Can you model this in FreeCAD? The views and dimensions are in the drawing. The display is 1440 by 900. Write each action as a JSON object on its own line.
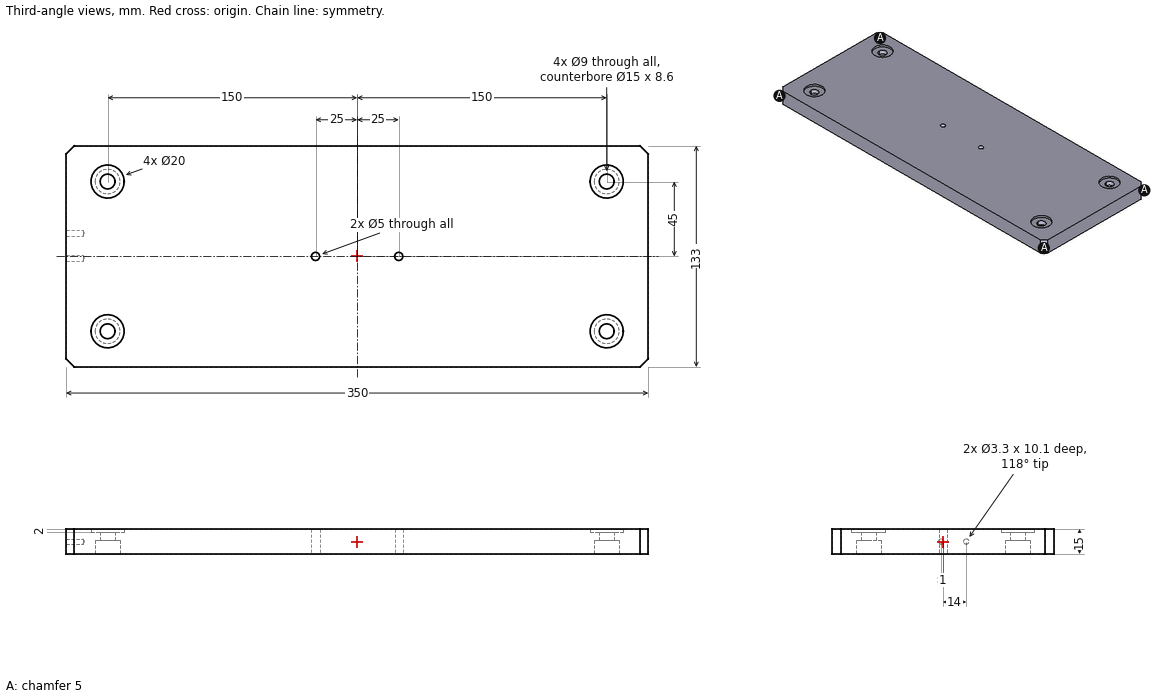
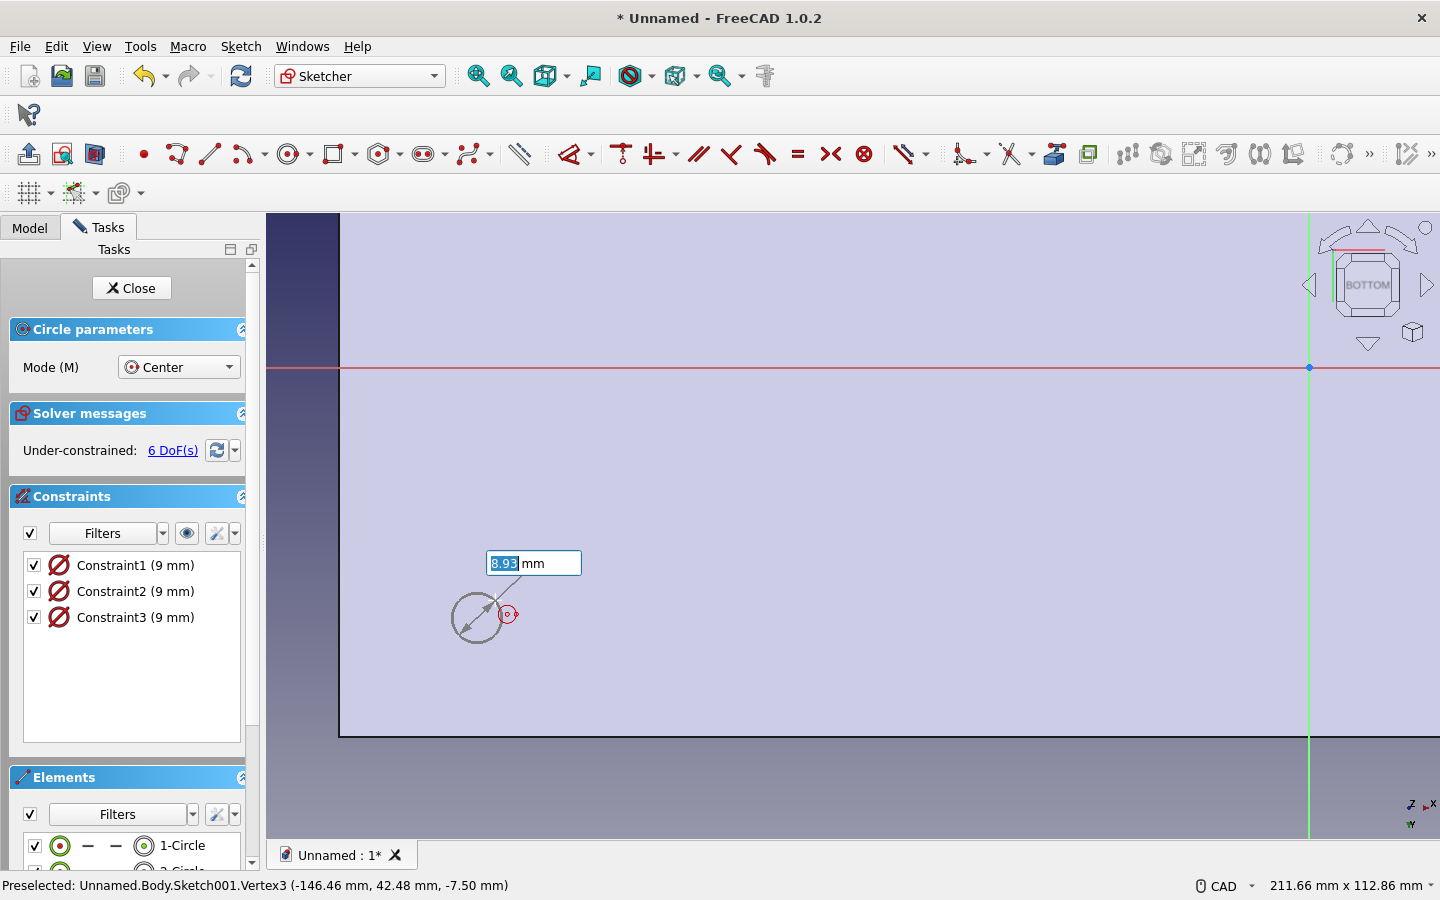
{"action": "type", "text": "9"}
{"action": "key", "text": "Return"}
{"action": "key", "text": "Escape"}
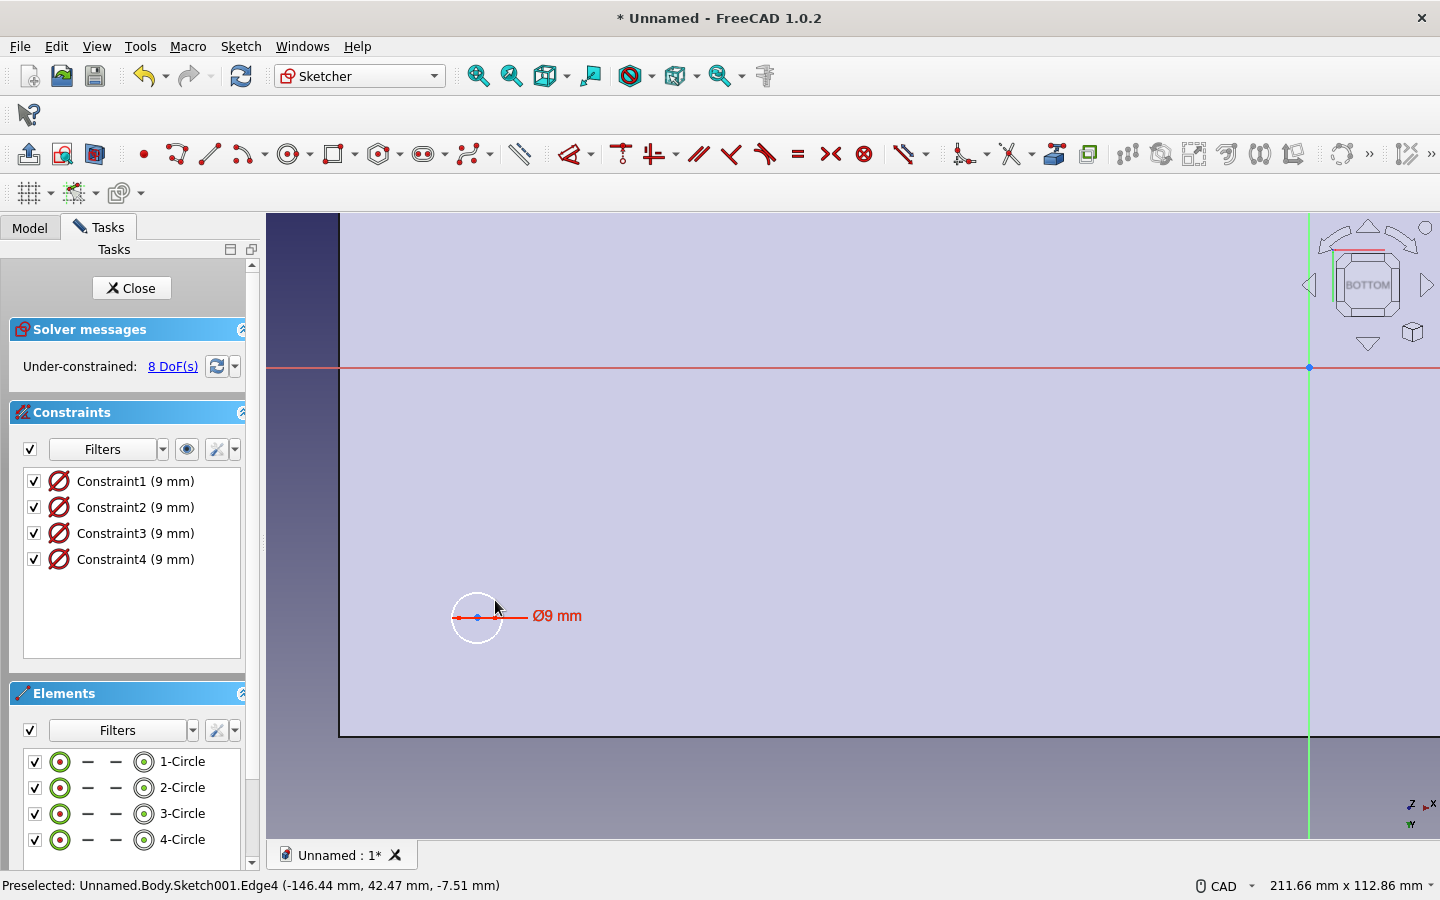
{"action": "scroll", "coordinate": [479, 618], "scroll_direction": "down", "scroll_amount": 5}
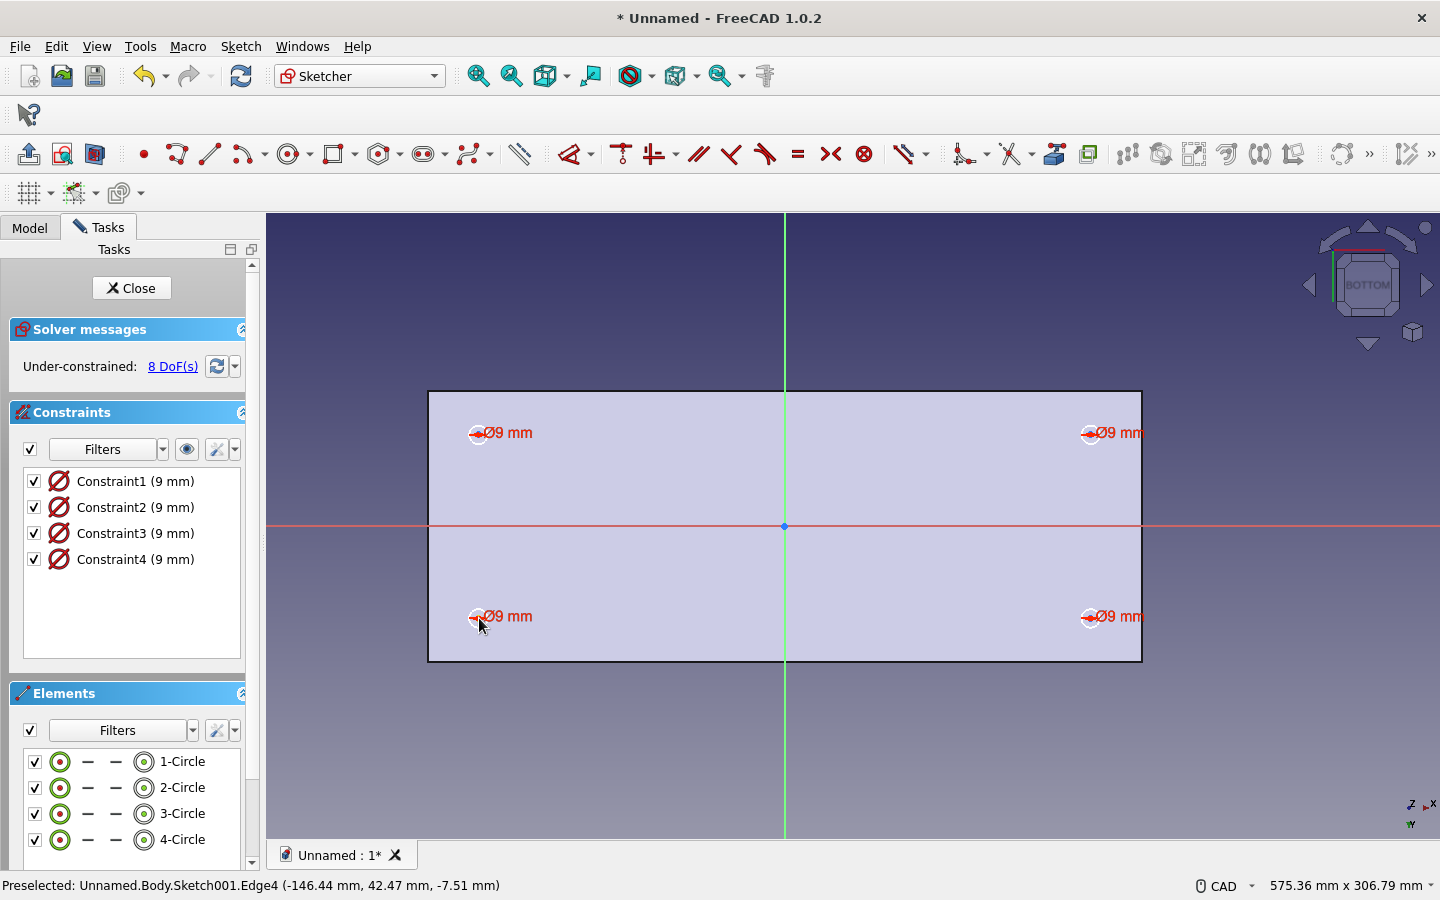
{"action": "left_click", "coordinate": [1091, 618]}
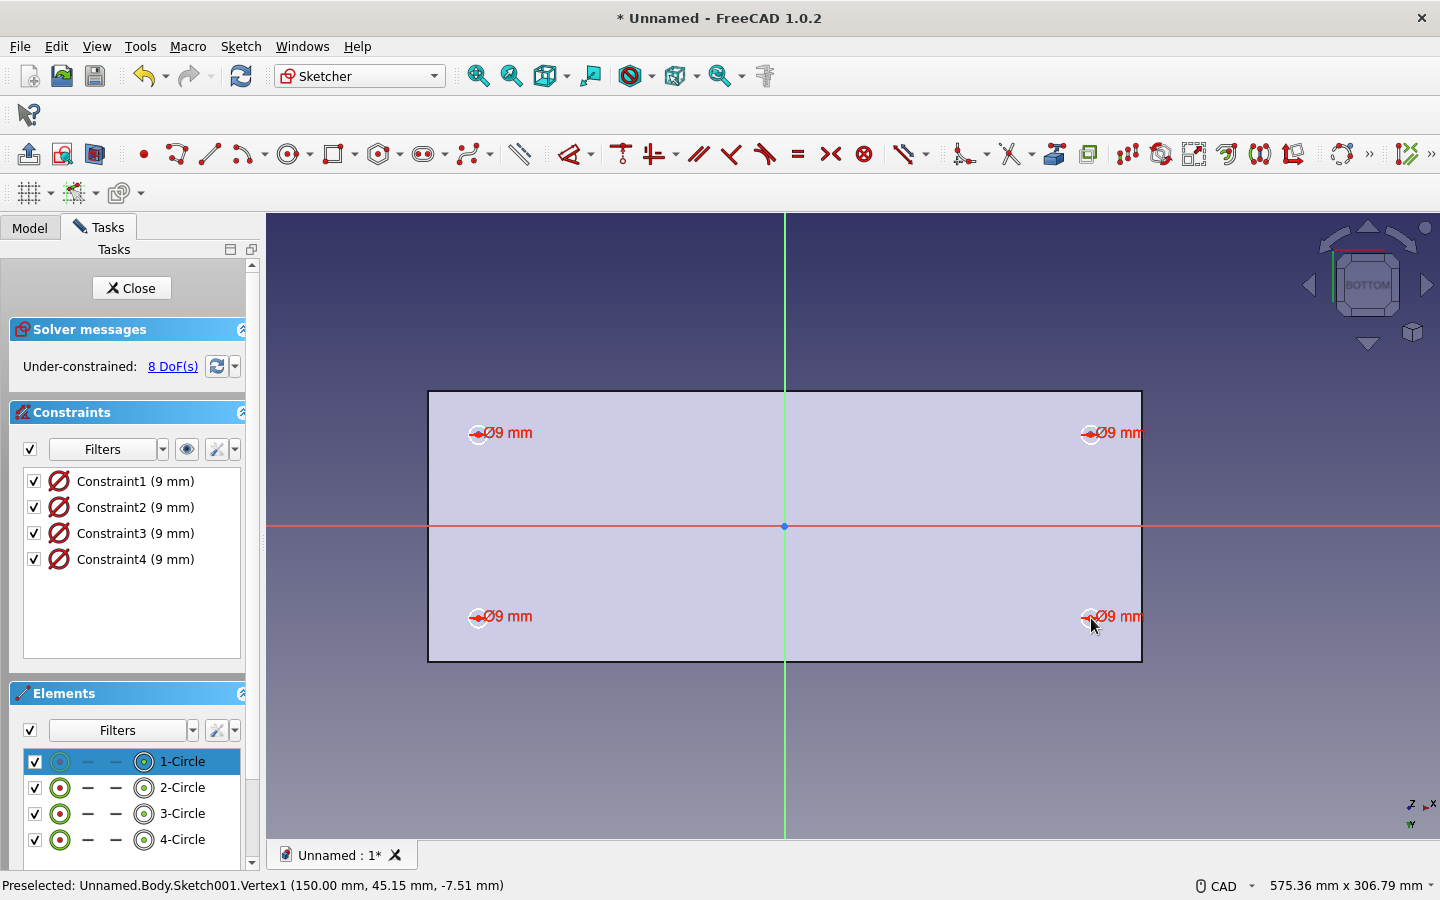
{"action": "left_click", "coordinate": [1091, 435]}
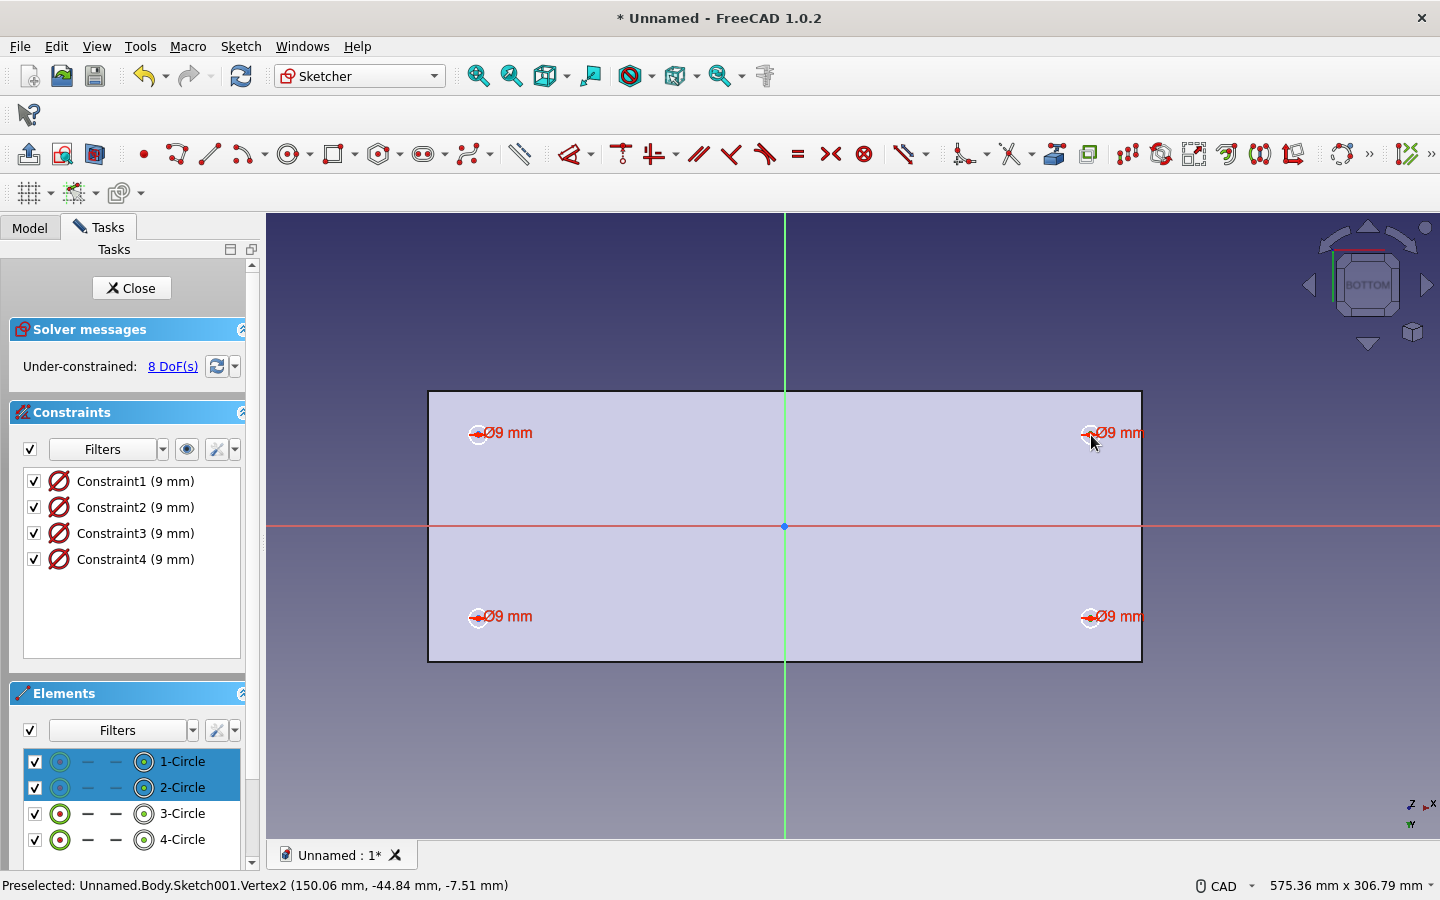
{"action": "left_click", "coordinate": [364, 526]}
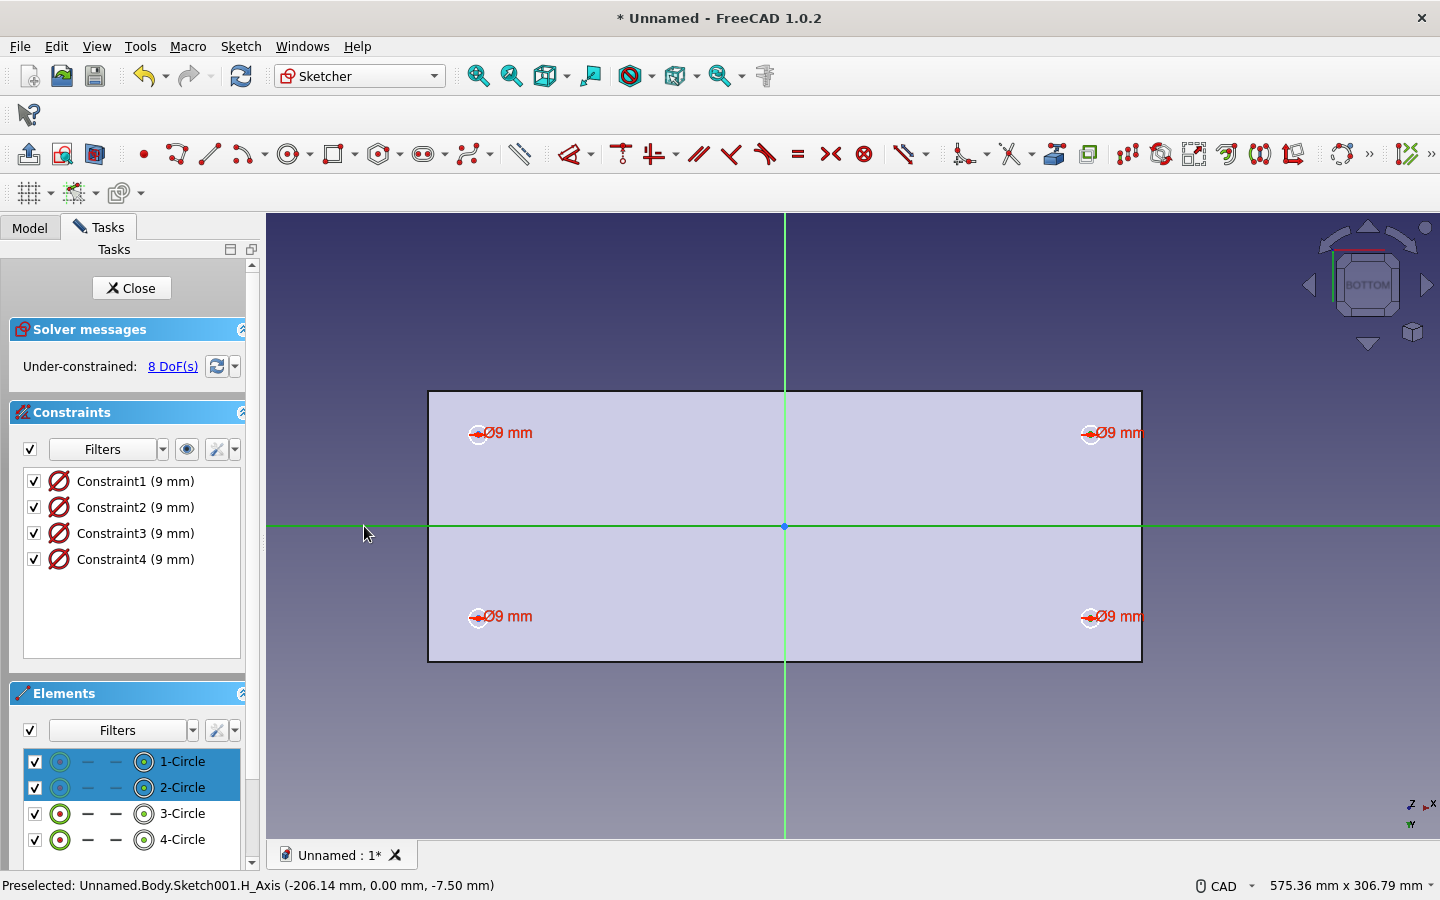
{"action": "key", "text": "s"}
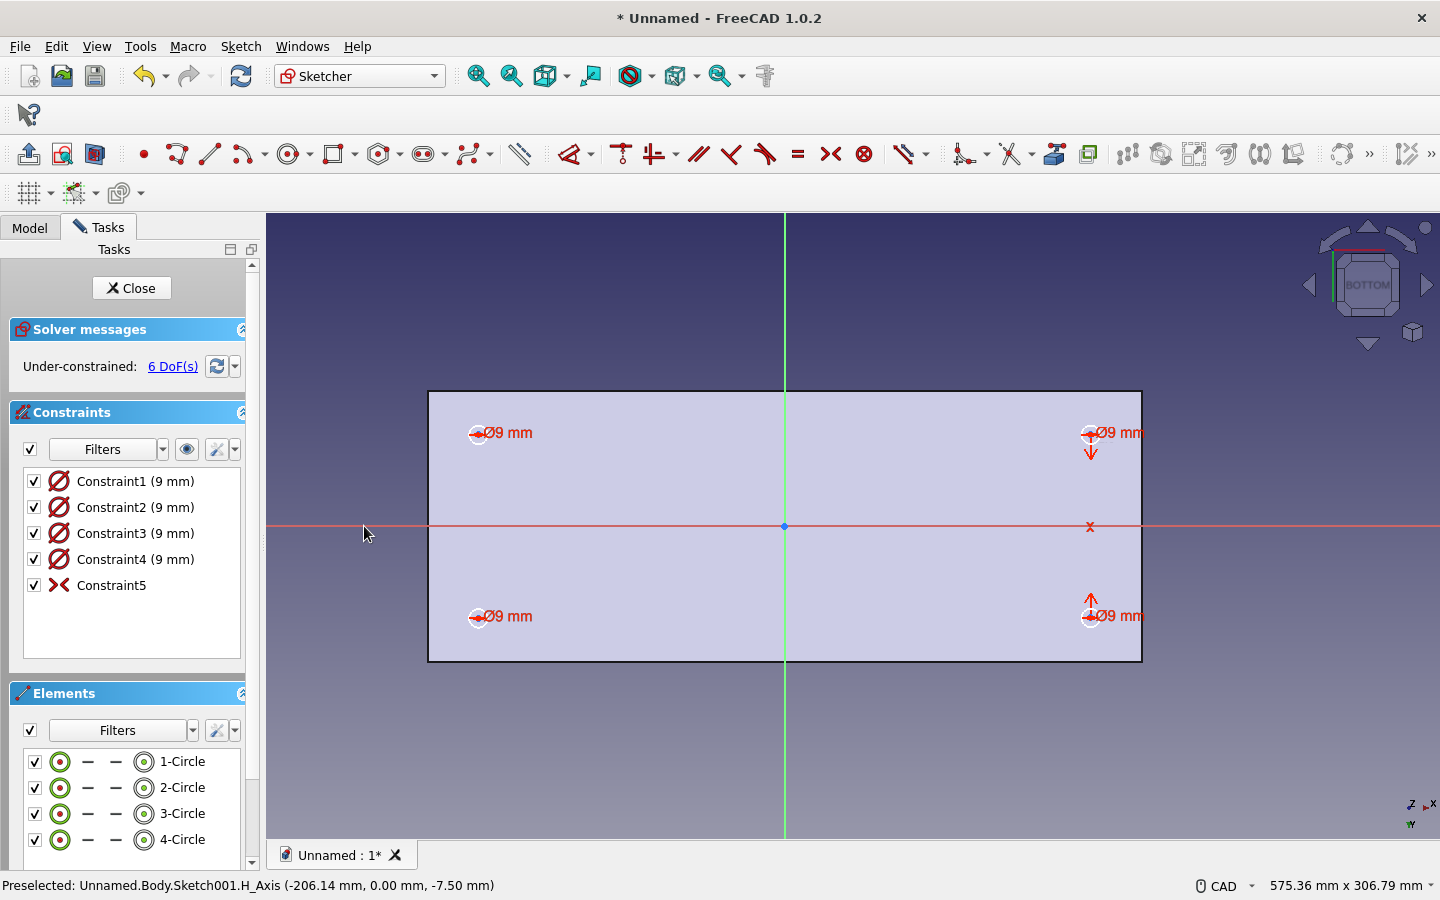
{"action": "left_click", "coordinate": [1091, 435]}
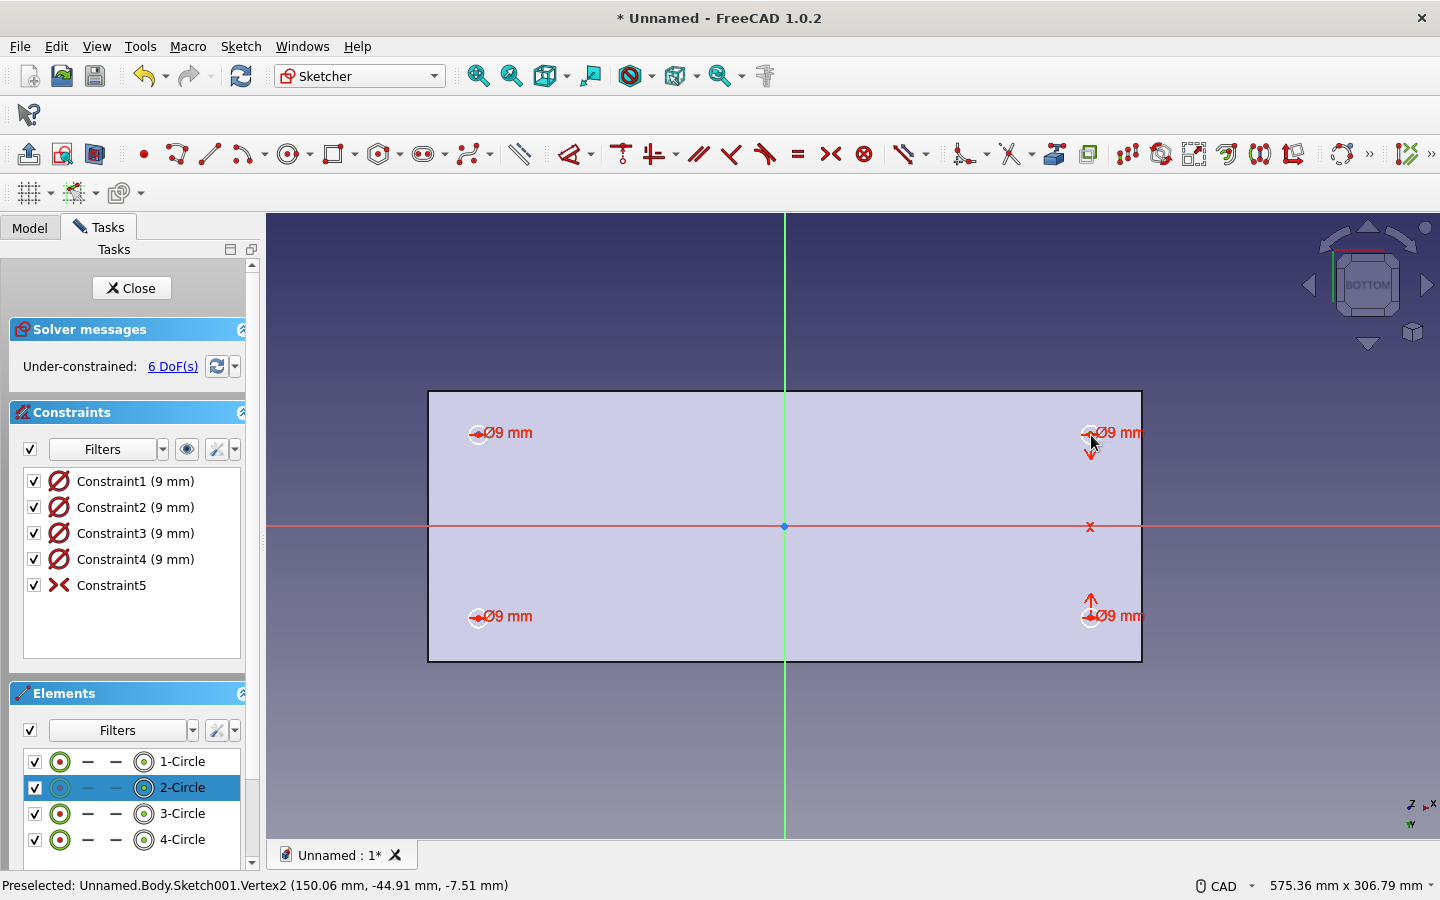
{"action": "left_click", "coordinate": [478, 435]}